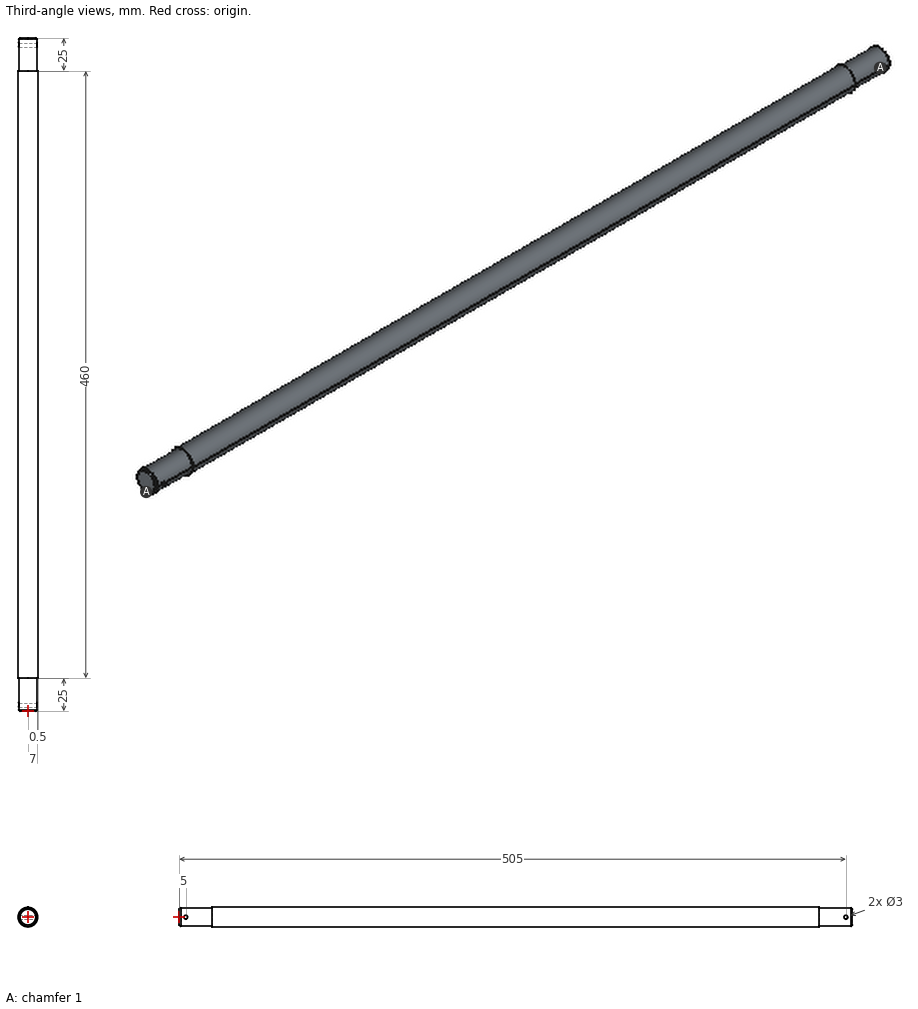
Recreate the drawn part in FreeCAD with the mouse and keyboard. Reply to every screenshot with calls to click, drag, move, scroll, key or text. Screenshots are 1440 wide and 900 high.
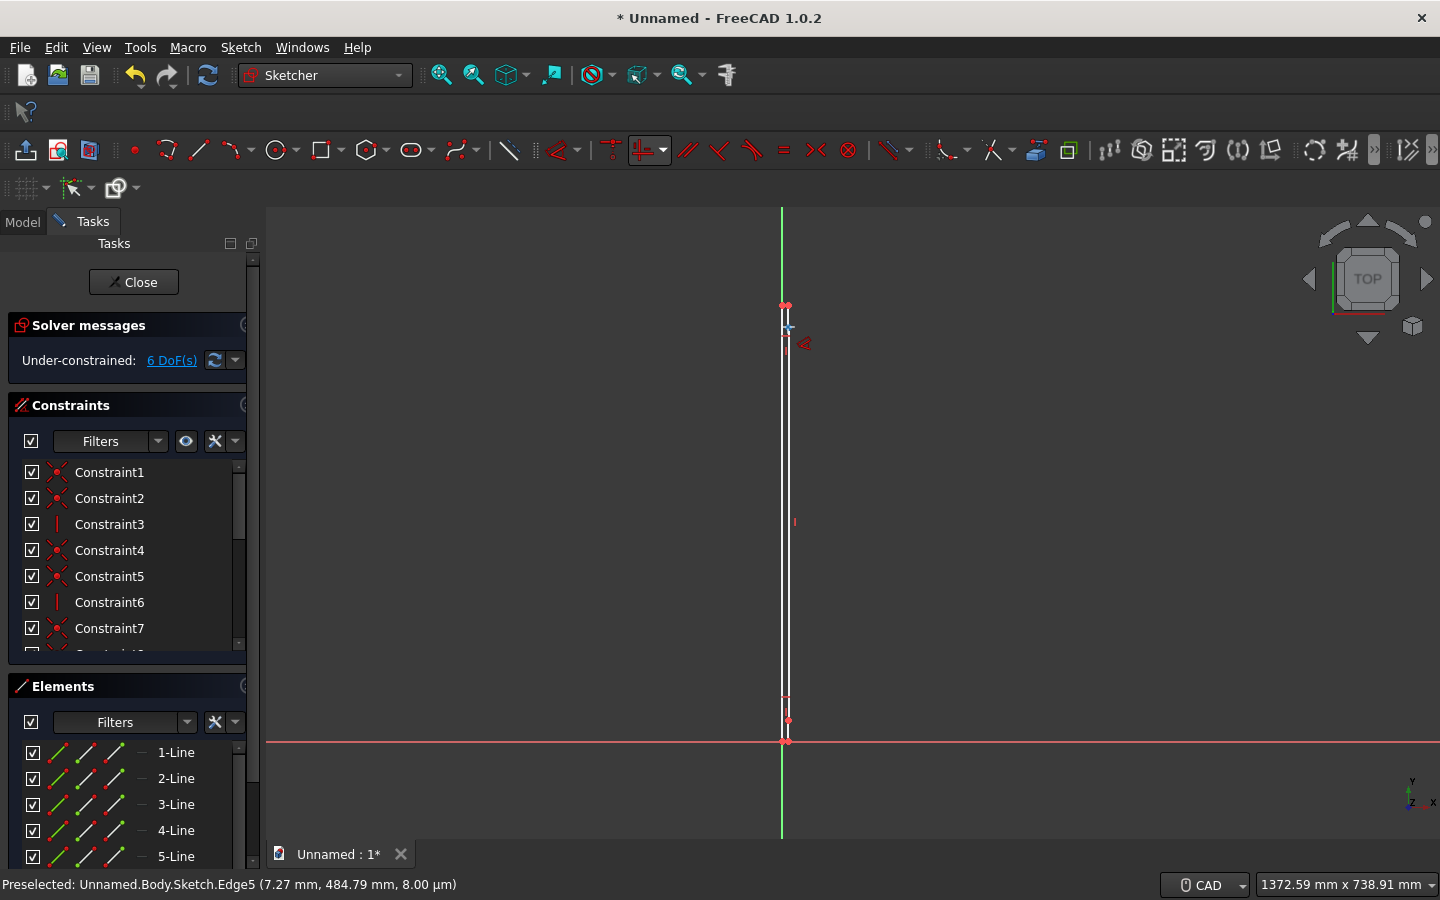
scroll(784, 742, up, 11)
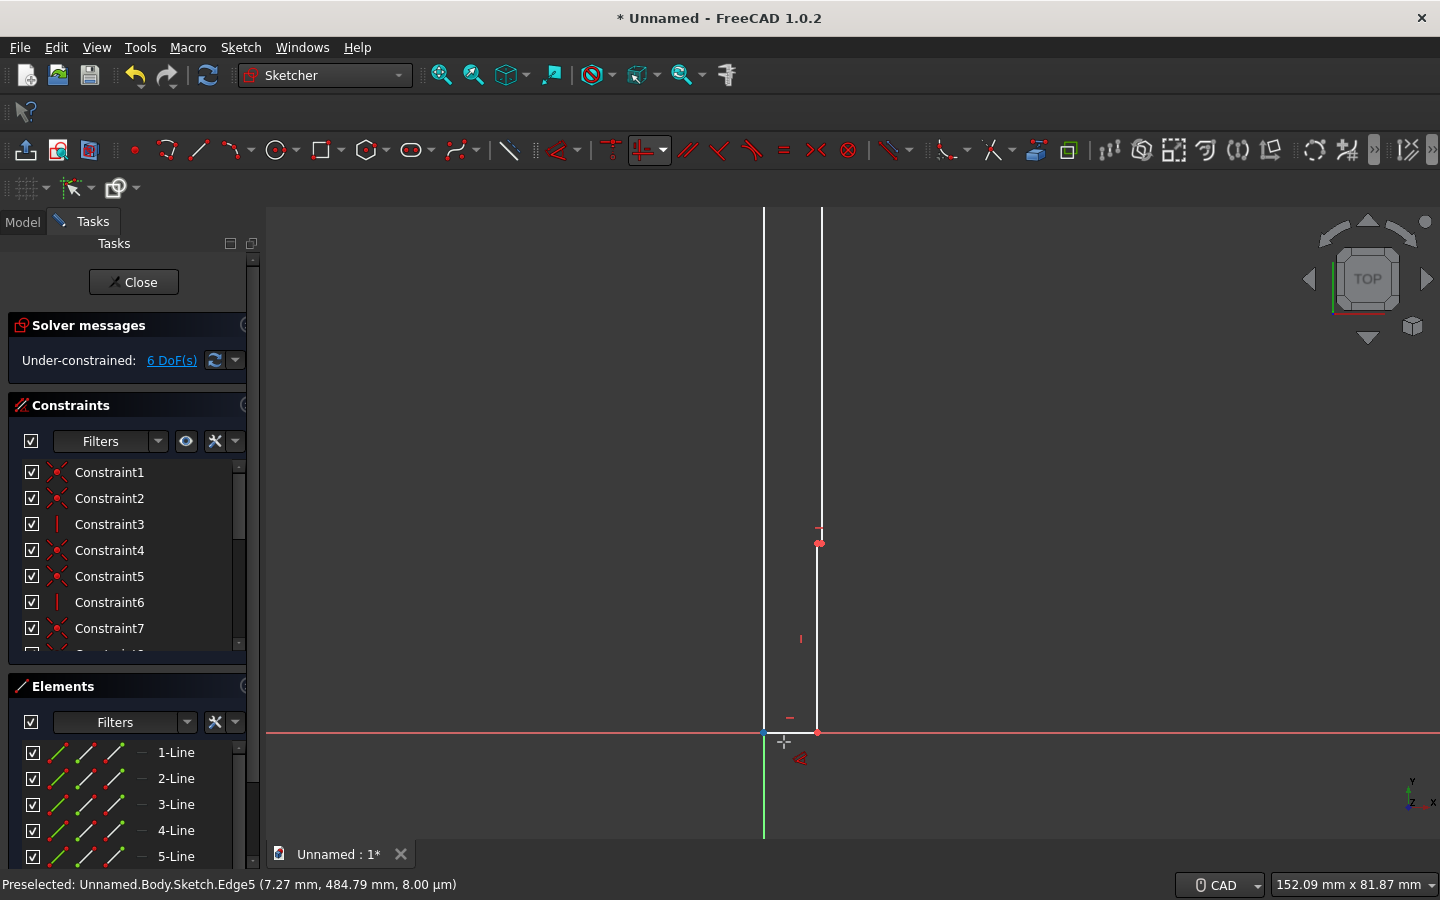
click(780, 733)
click(790, 767)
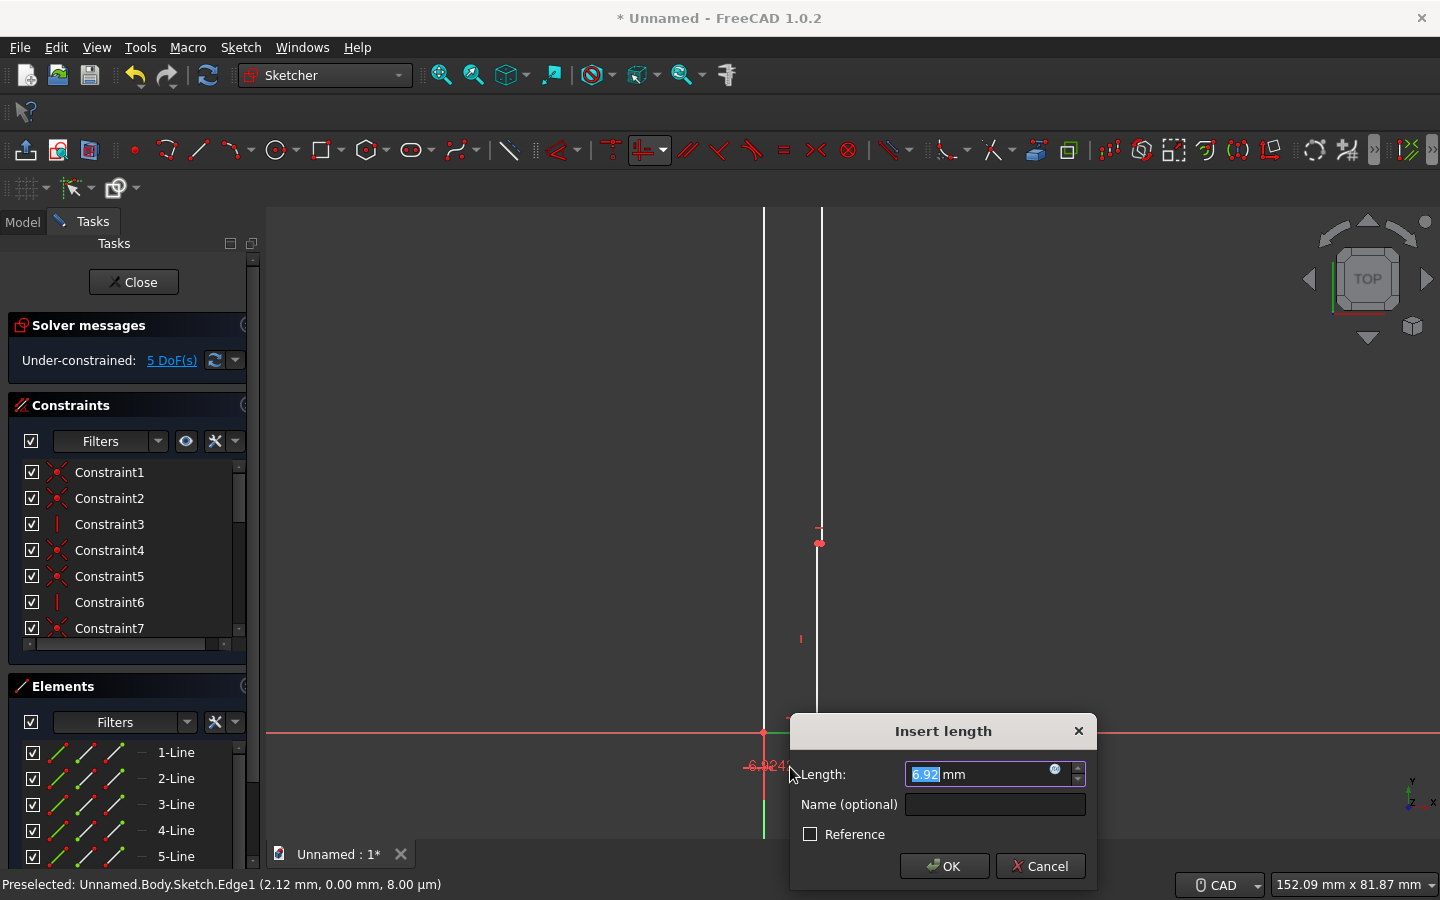
text(7)
key(Return)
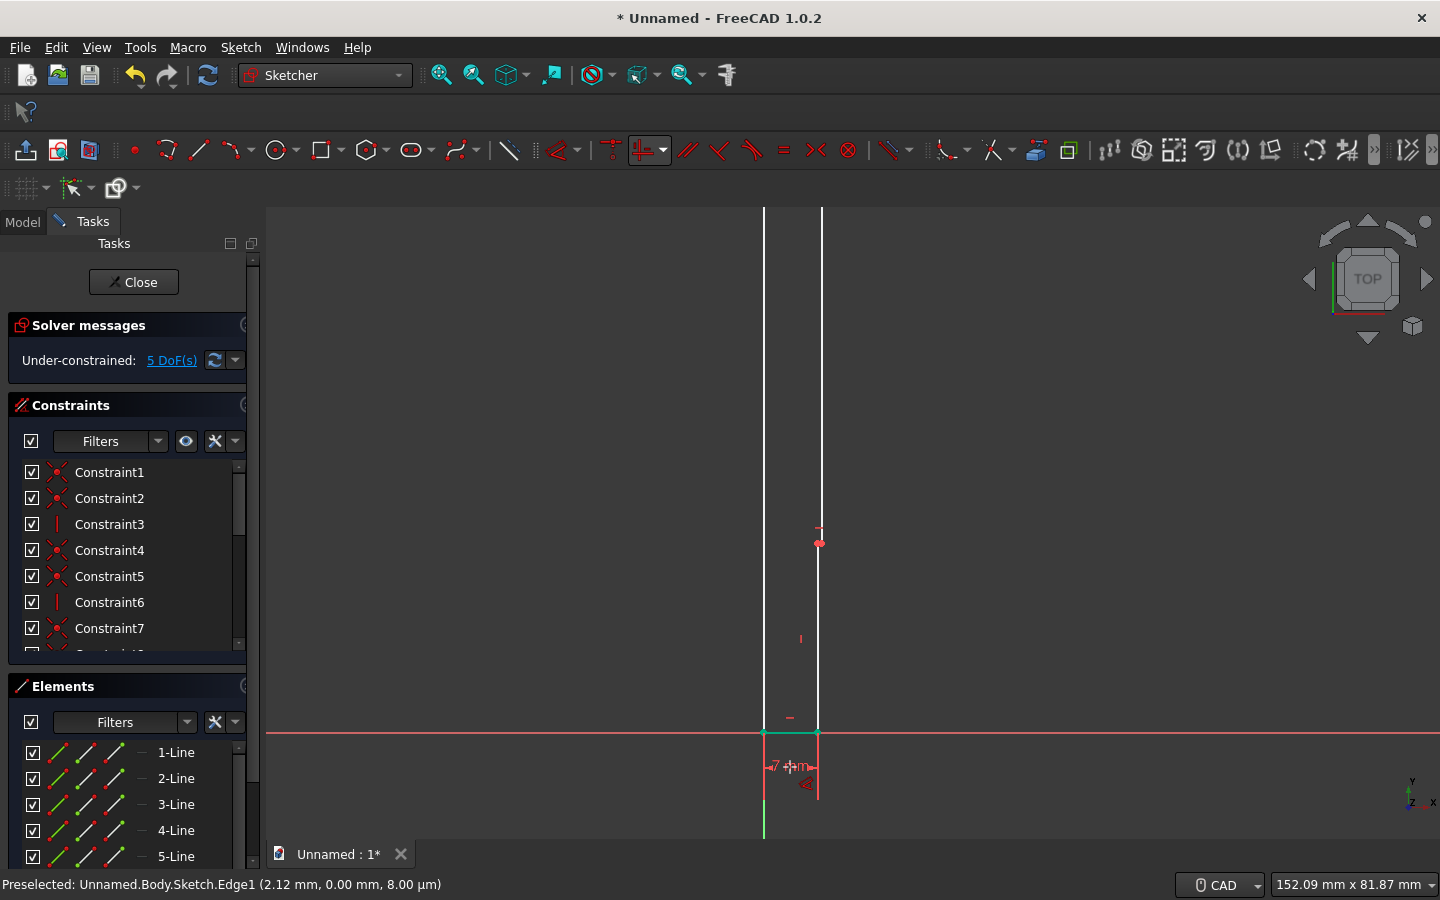
scroll(783, 742, down, 11)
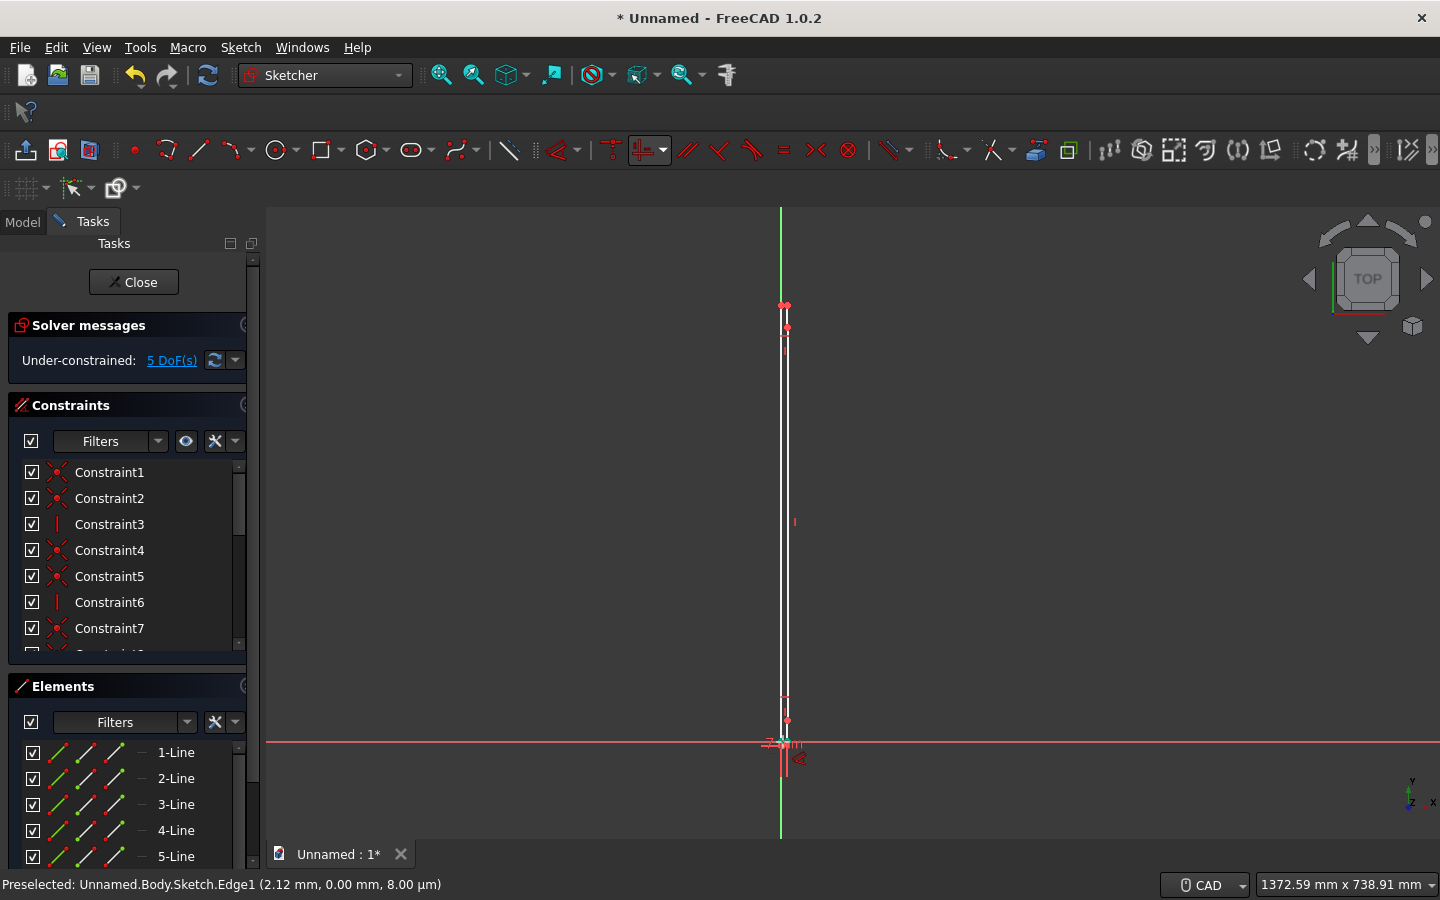
scroll(785, 306, up, 11)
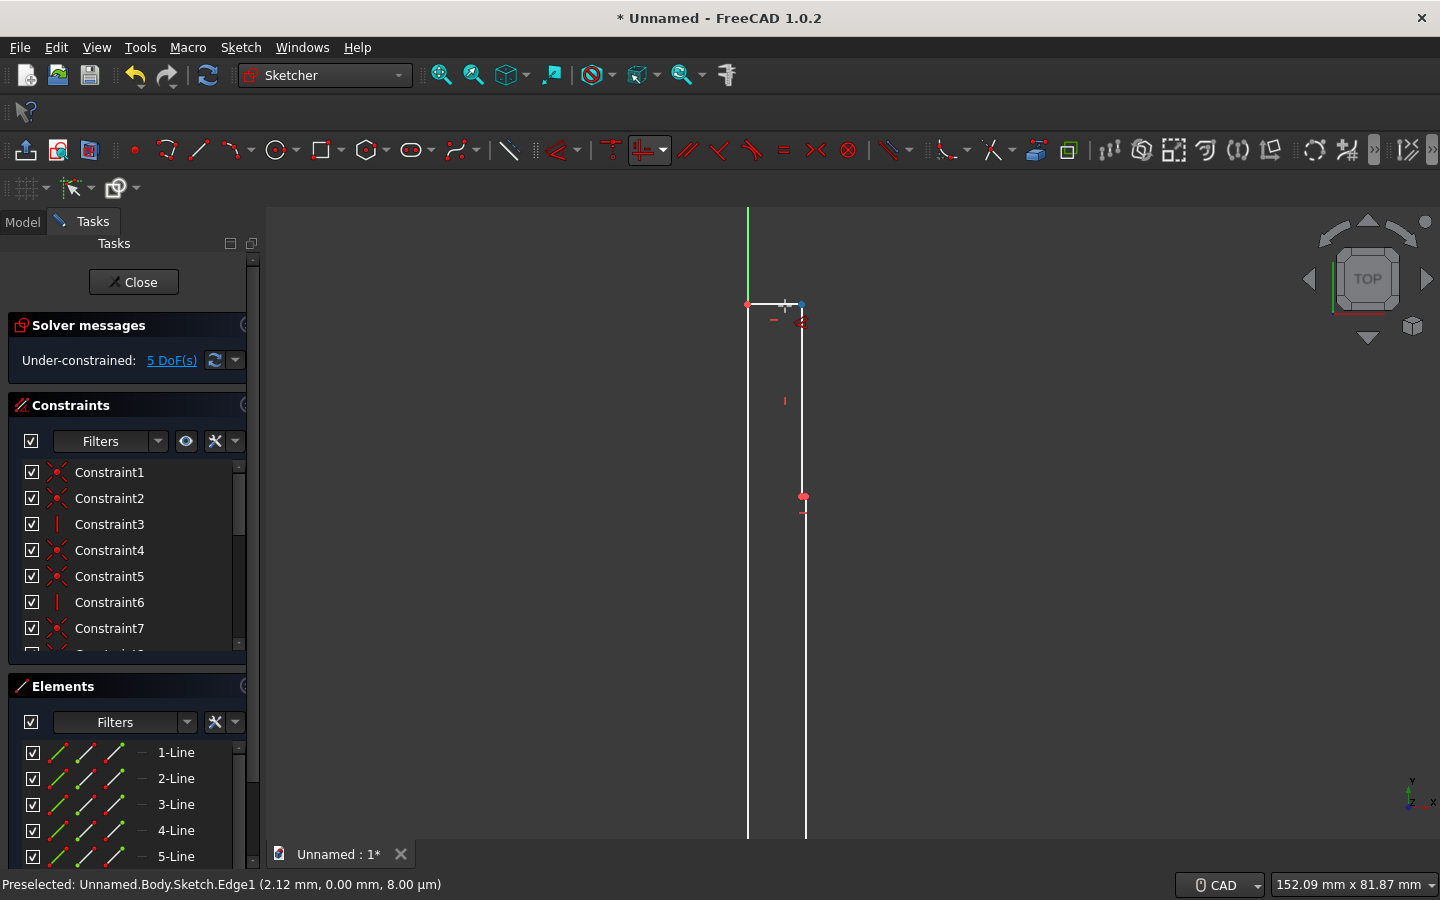
click(785, 304)
click(775, 270)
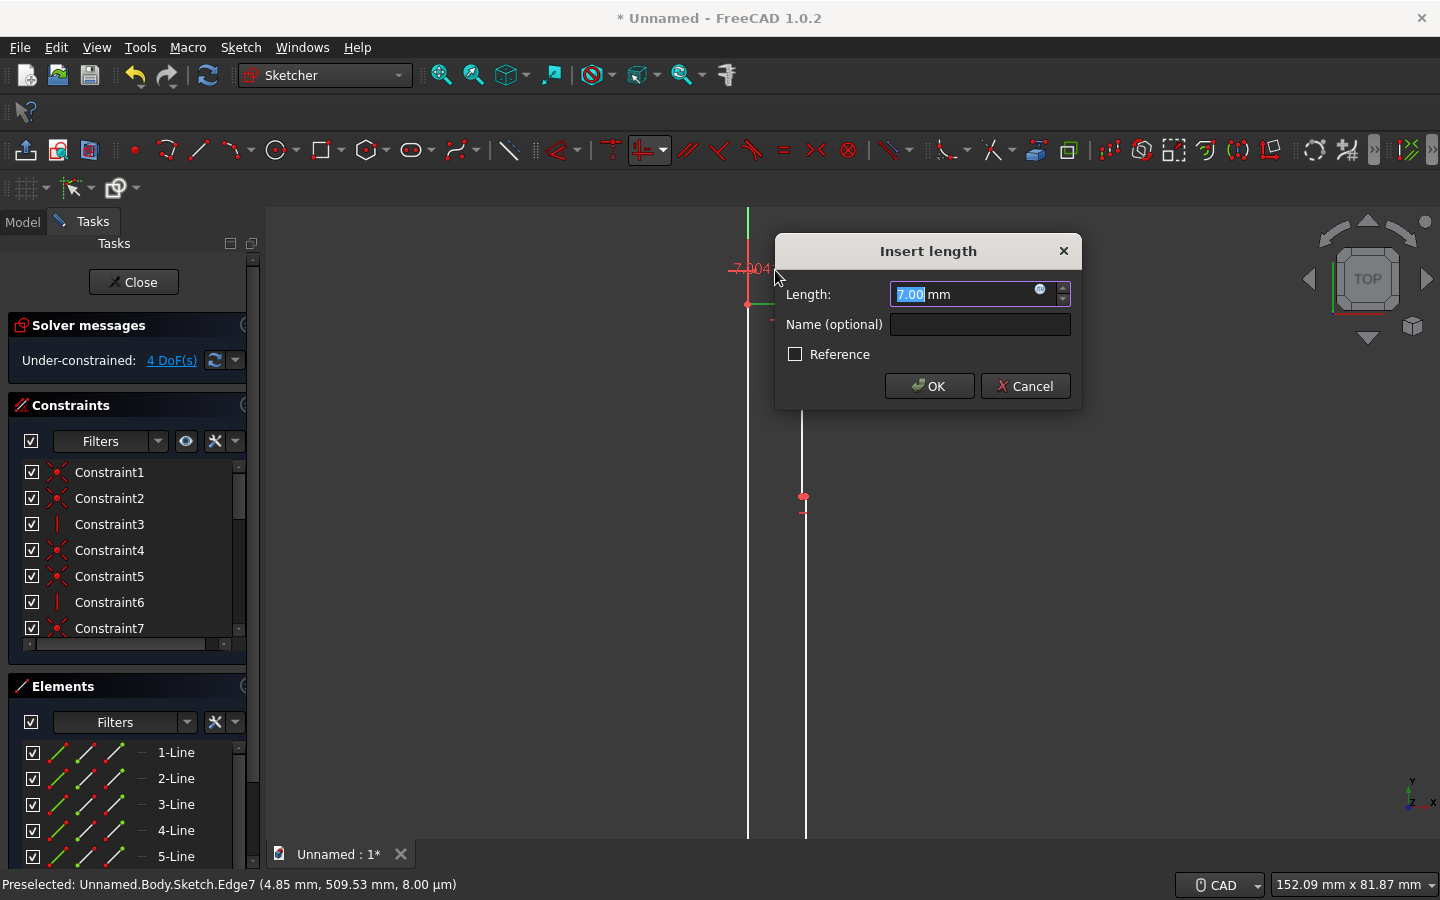
text(7)
key(Return)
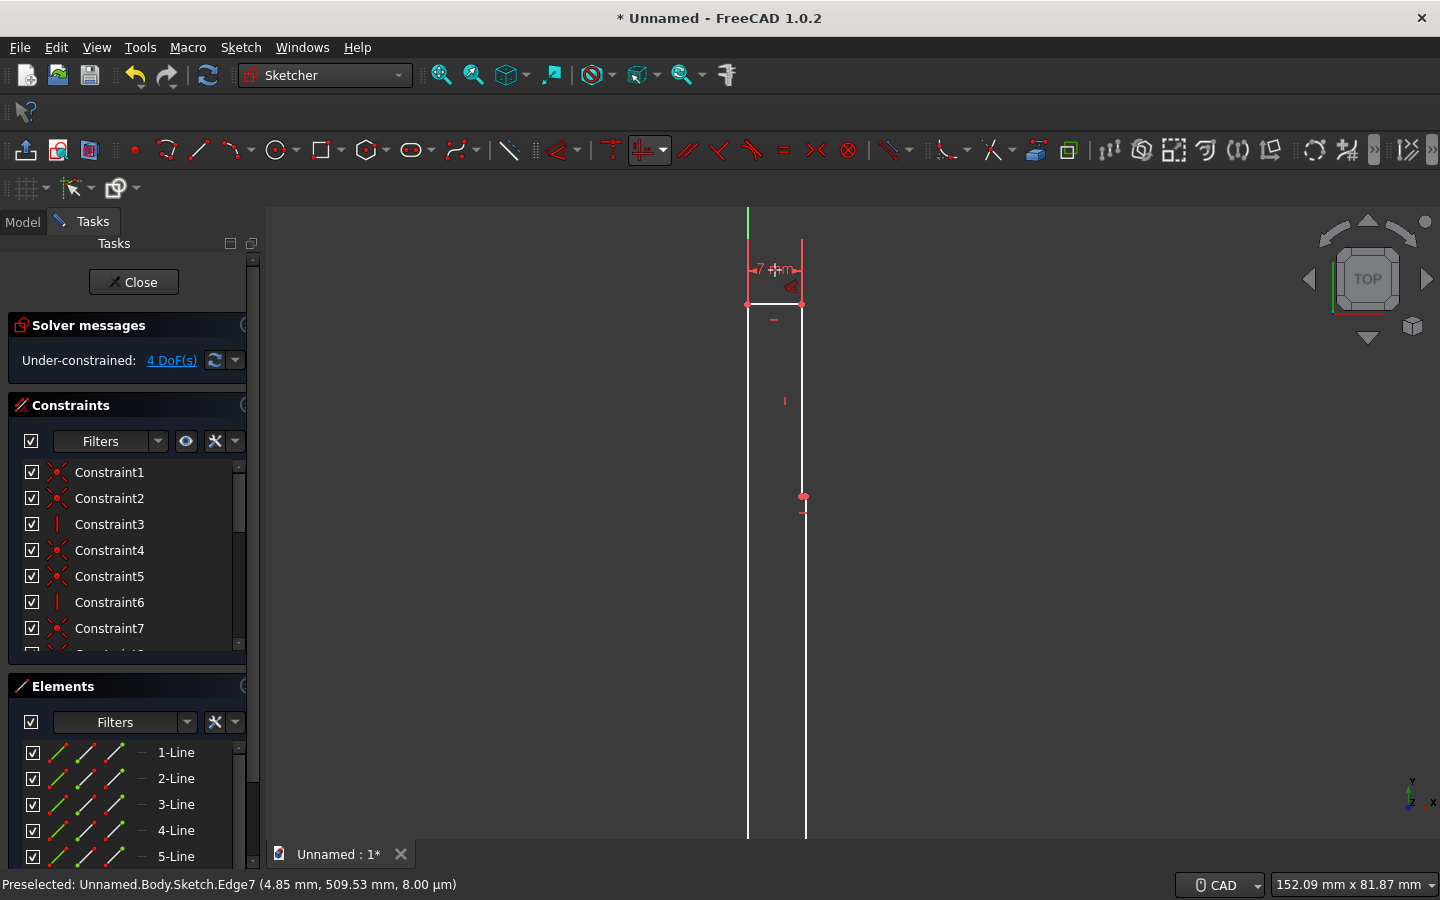
scroll(785, 305, down, 11)